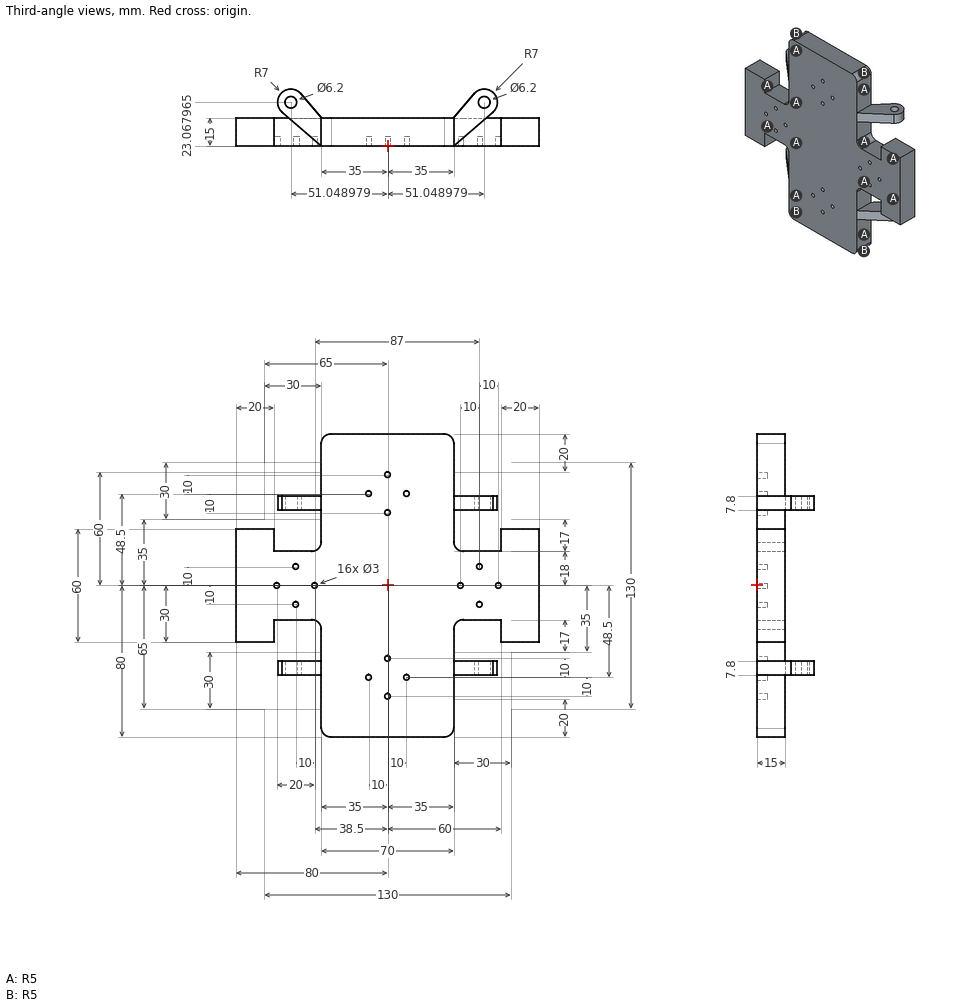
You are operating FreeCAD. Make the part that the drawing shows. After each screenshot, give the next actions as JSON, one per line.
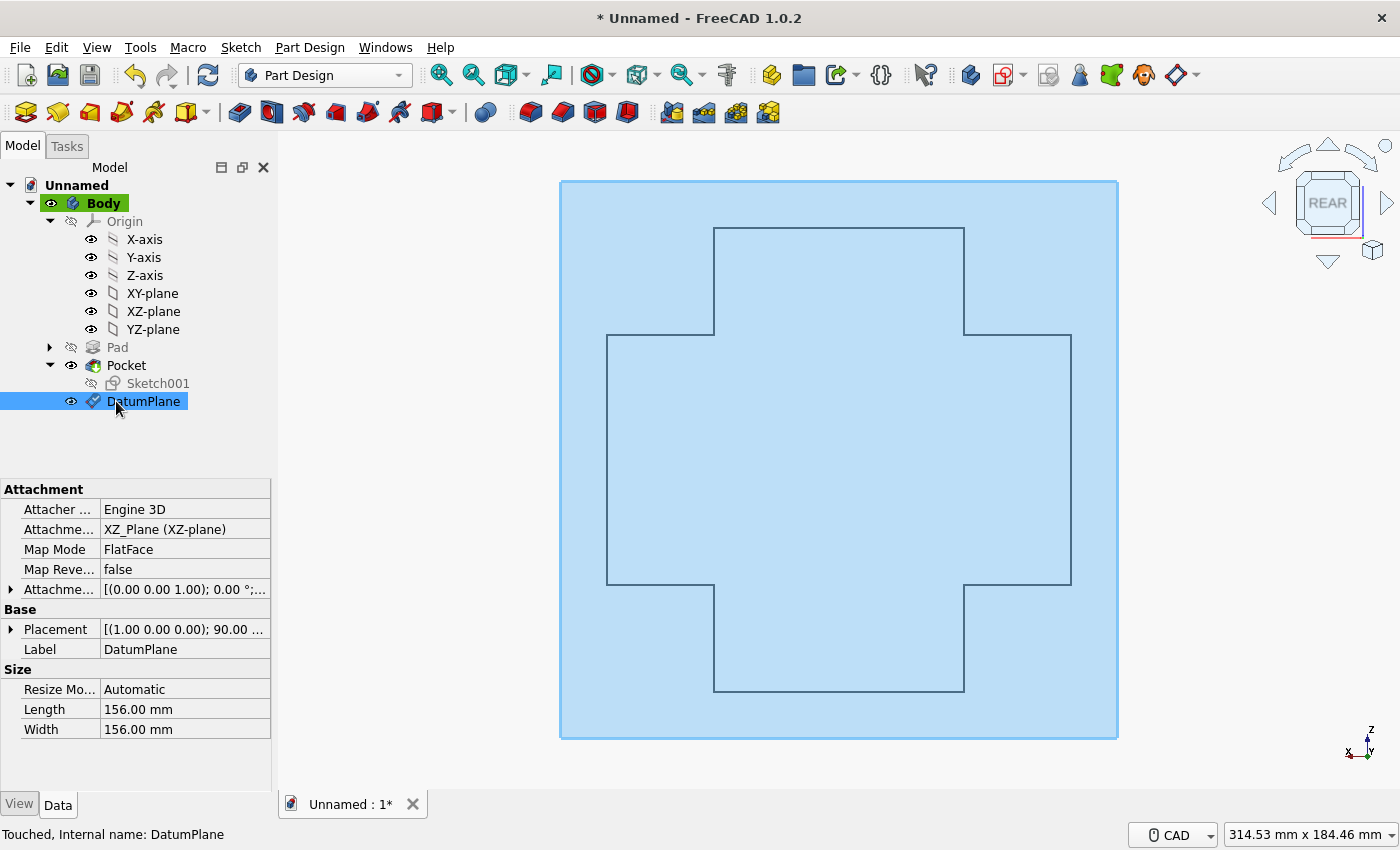
{"action": "left_click", "coordinate": [1004, 76]}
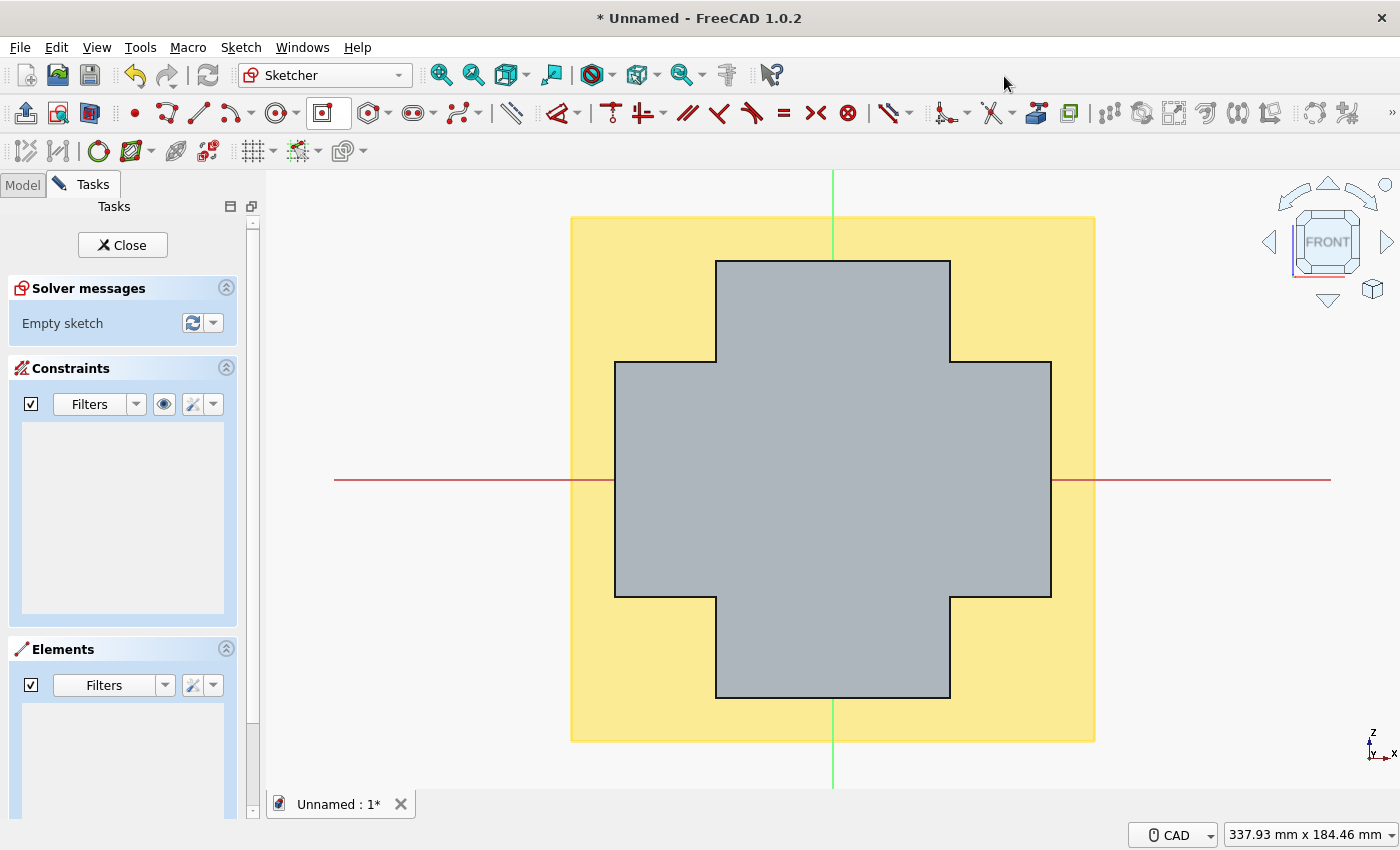
{"action": "left_click", "coordinate": [90, 114]}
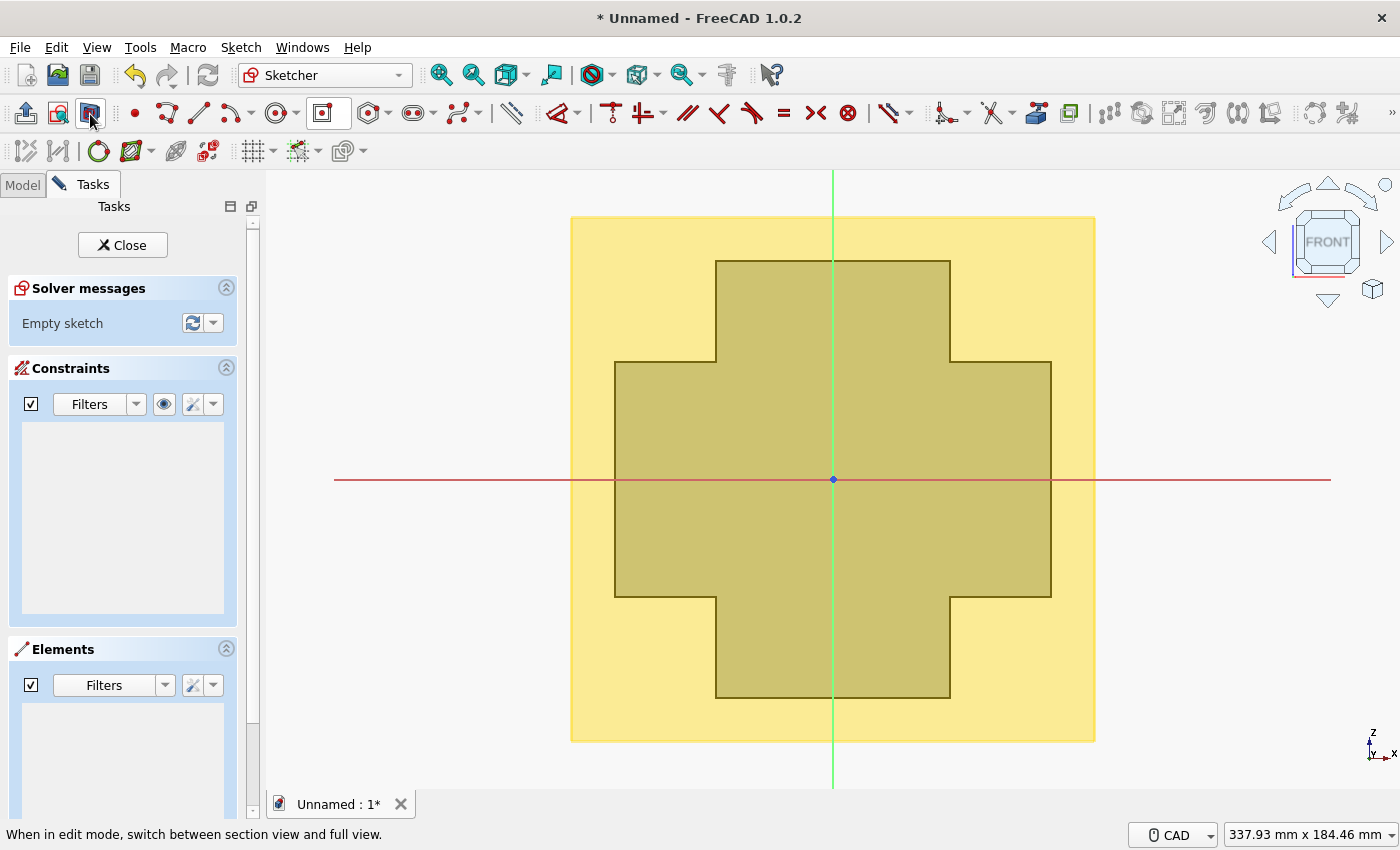
{"action": "left_click", "coordinate": [276, 114]}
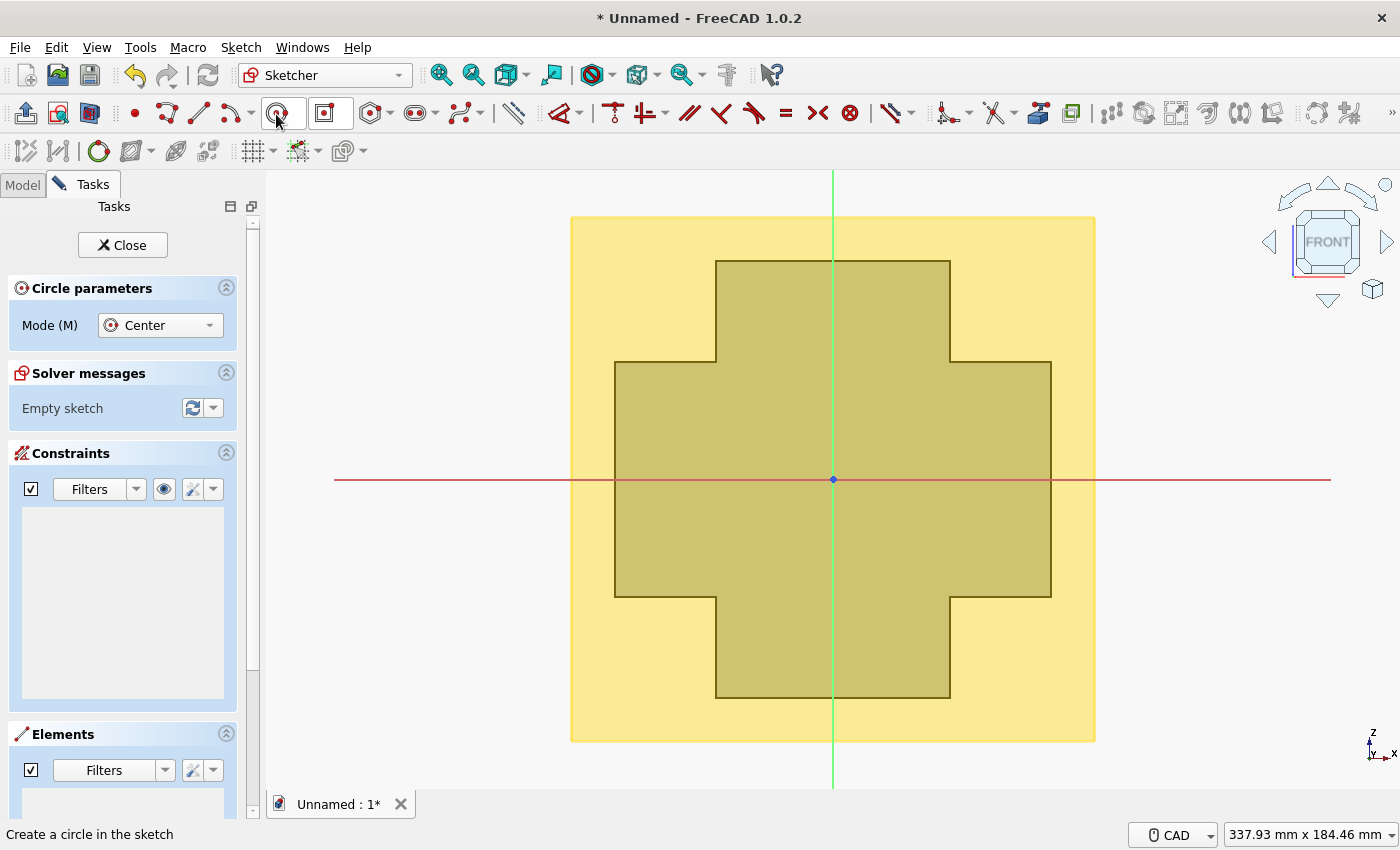
{"action": "scroll", "coordinate": [704, 480], "scroll_direction": "up", "scroll_amount": 8}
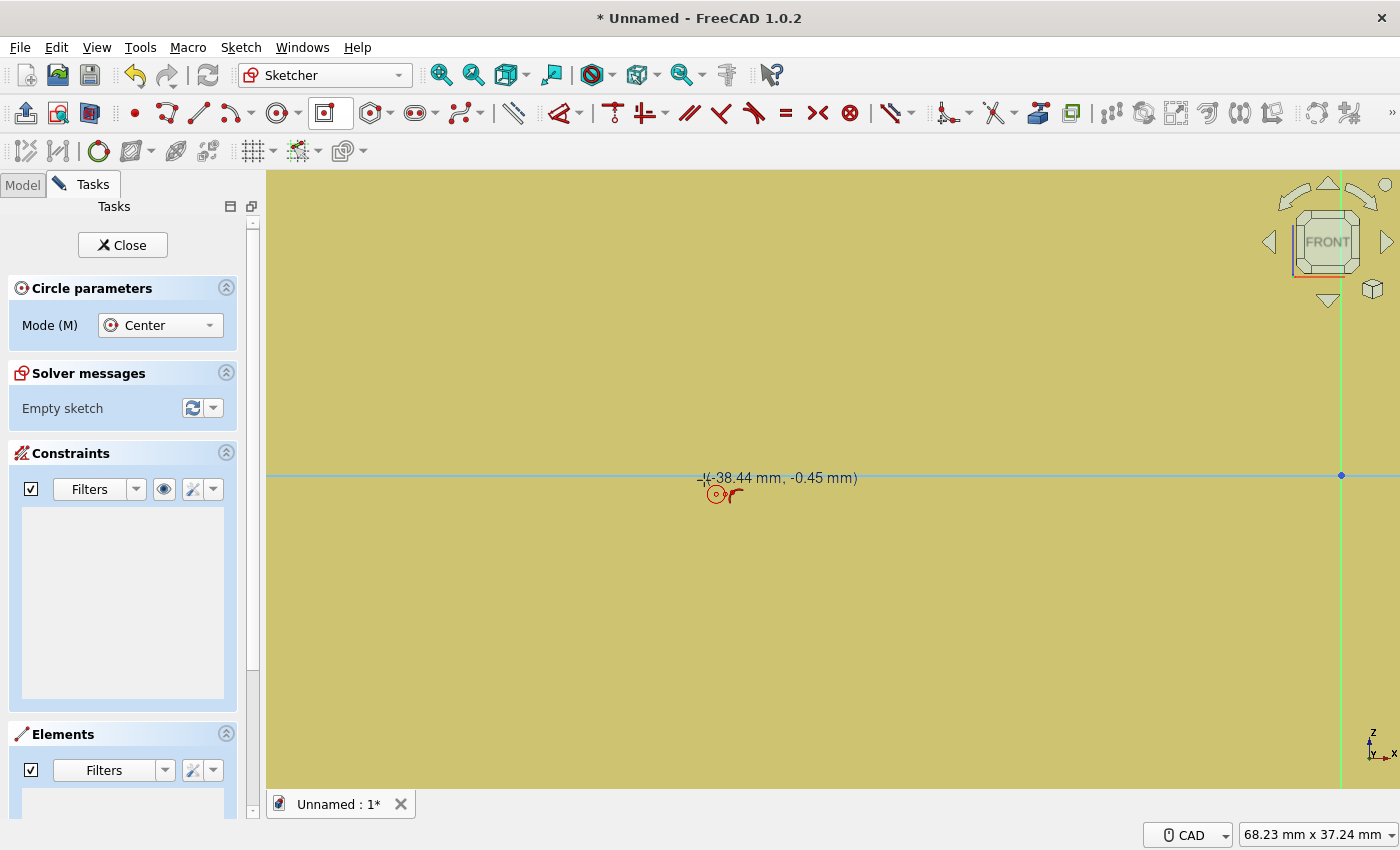
{"action": "scroll", "coordinate": [619, 481], "scroll_direction": "down", "scroll_amount": 8}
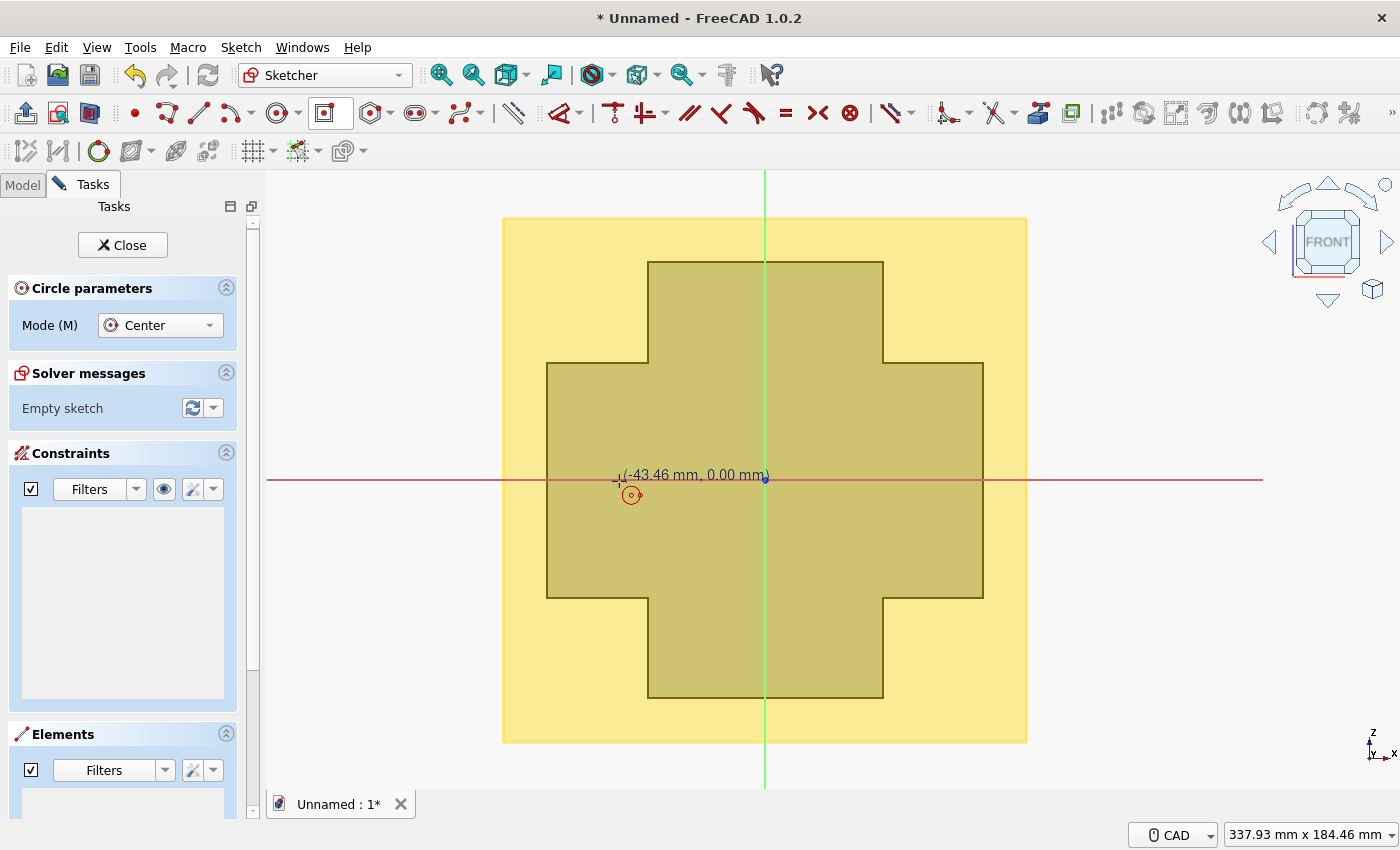
{"action": "left_click", "coordinate": [636, 480]}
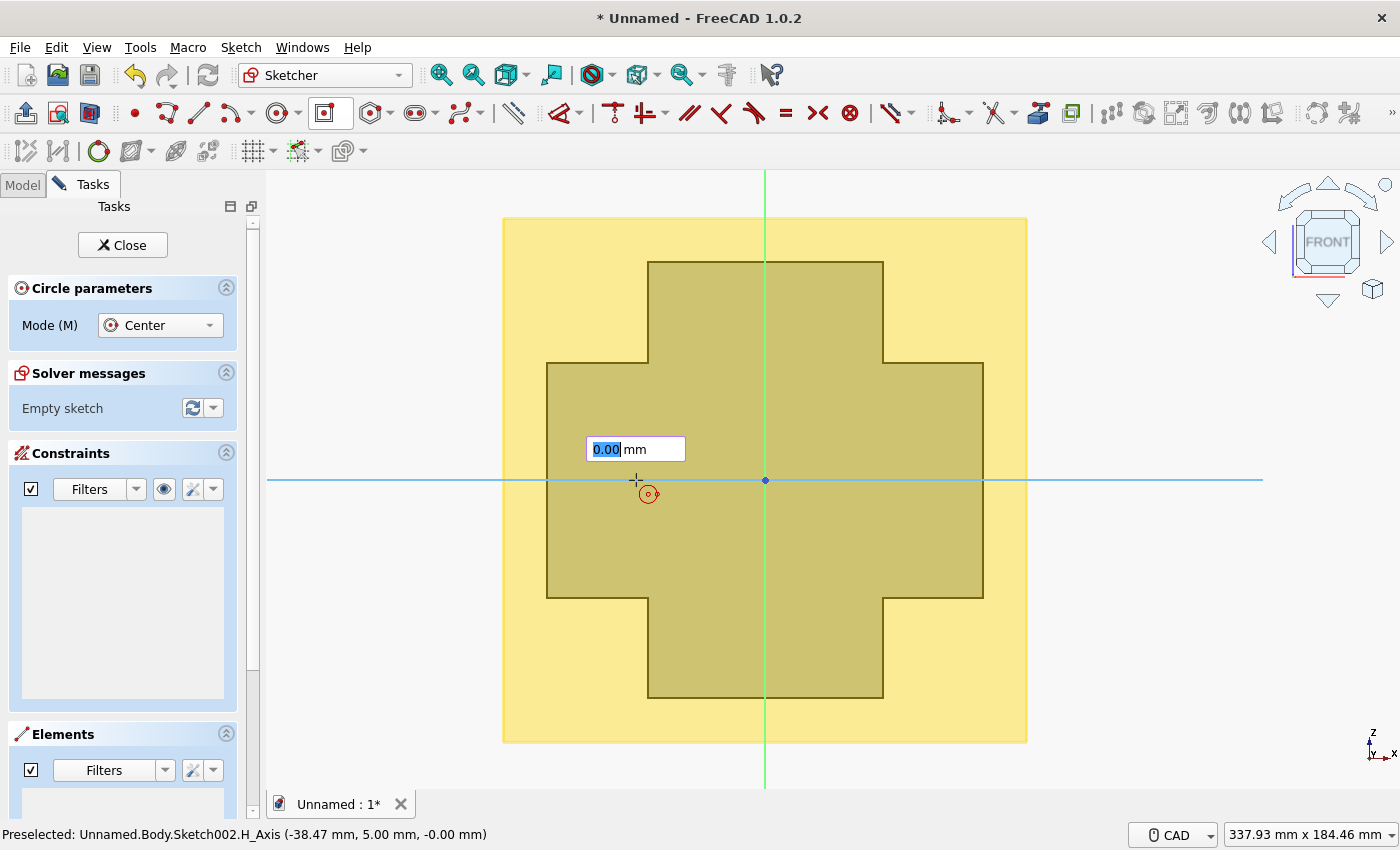
{"action": "scroll", "coordinate": [634, 485], "scroll_direction": "up", "scroll_amount": 7}
{"action": "mouse_move", "coordinate": [634, 484]}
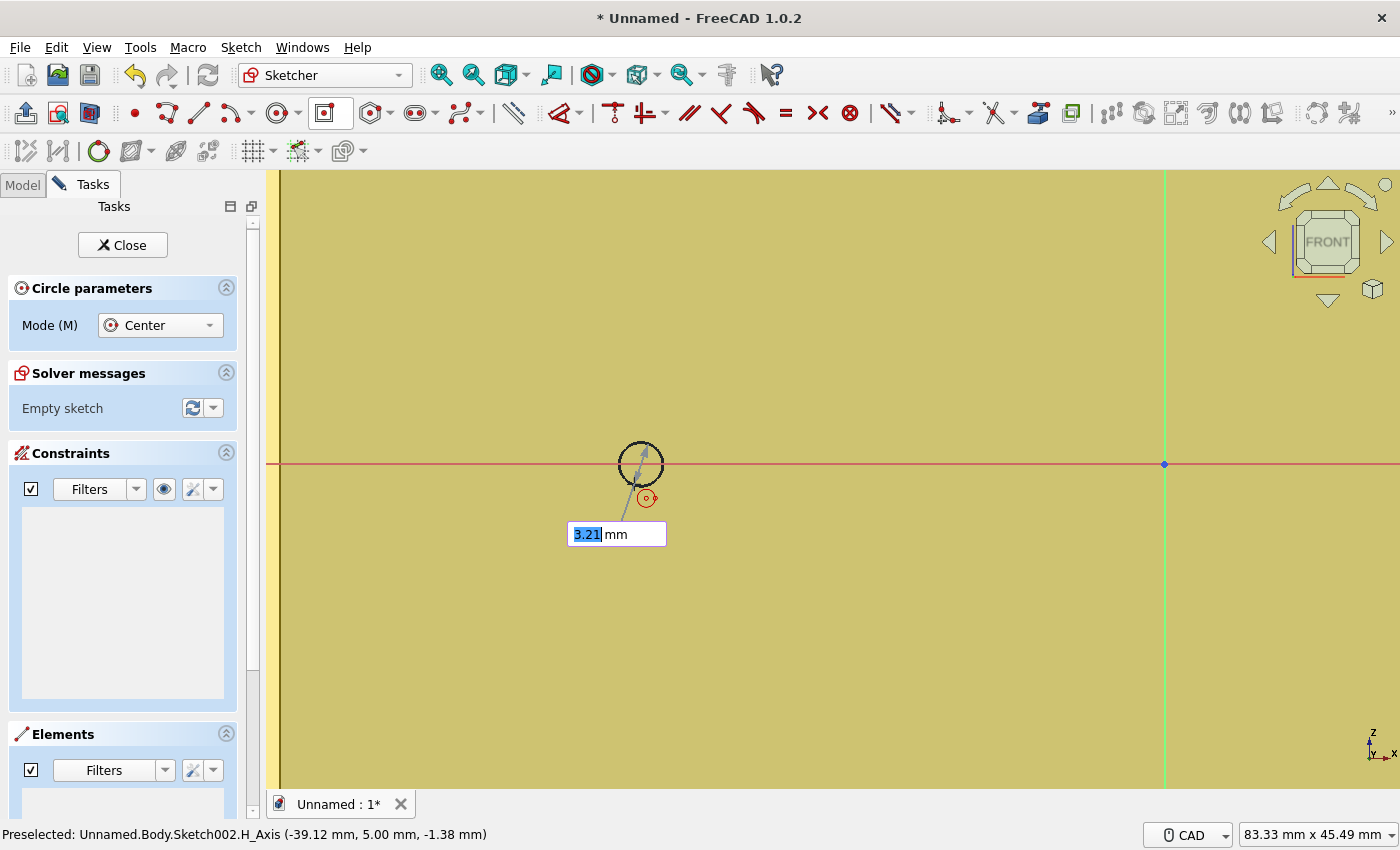
{"action": "type", "text": "3"}
{"action": "key", "text": "Return"}